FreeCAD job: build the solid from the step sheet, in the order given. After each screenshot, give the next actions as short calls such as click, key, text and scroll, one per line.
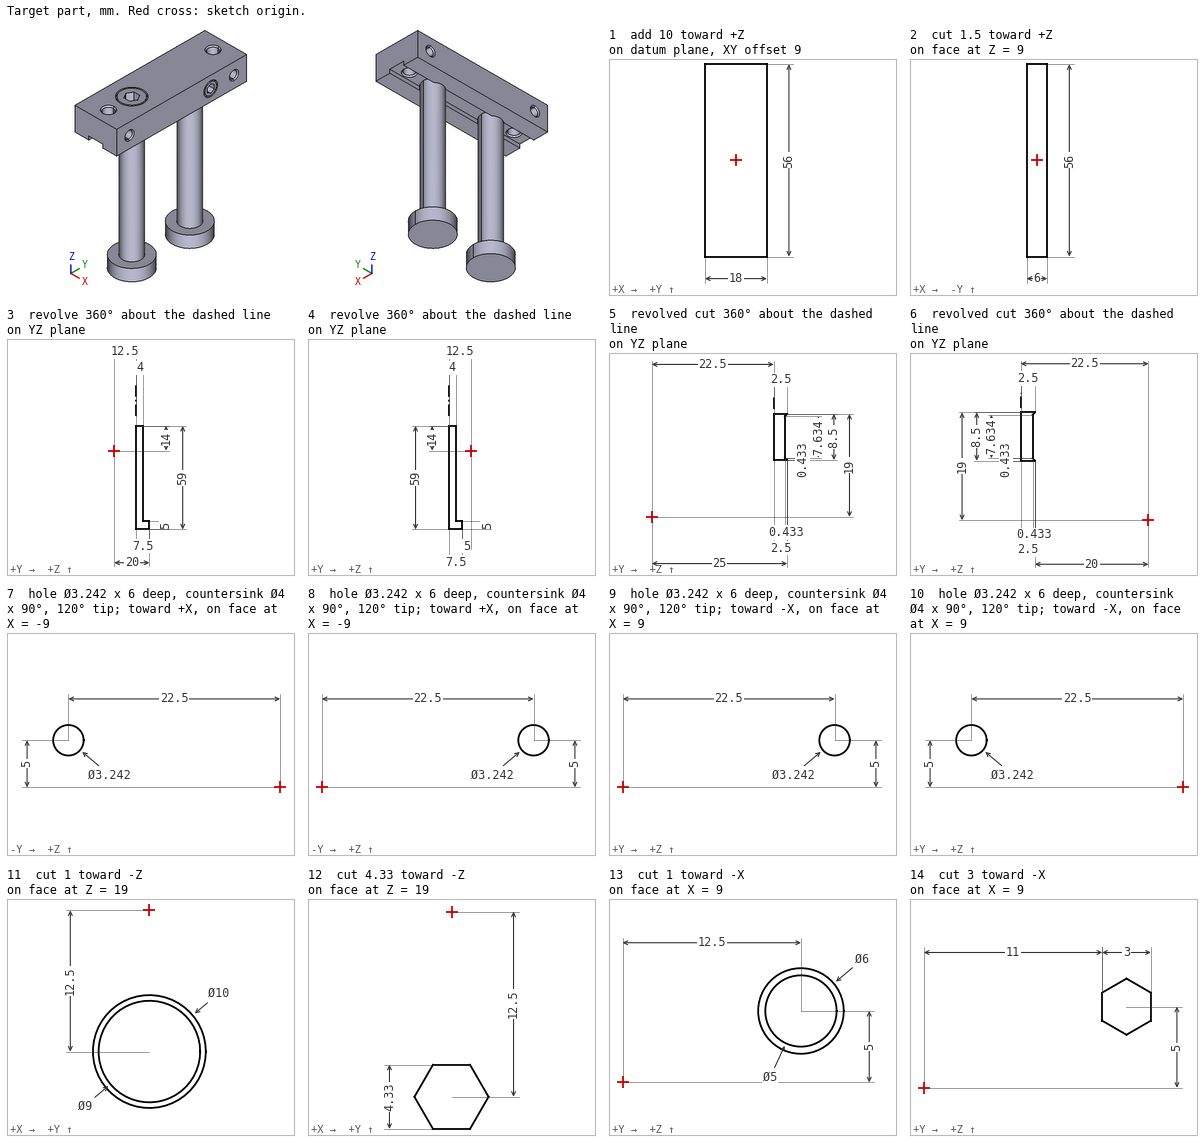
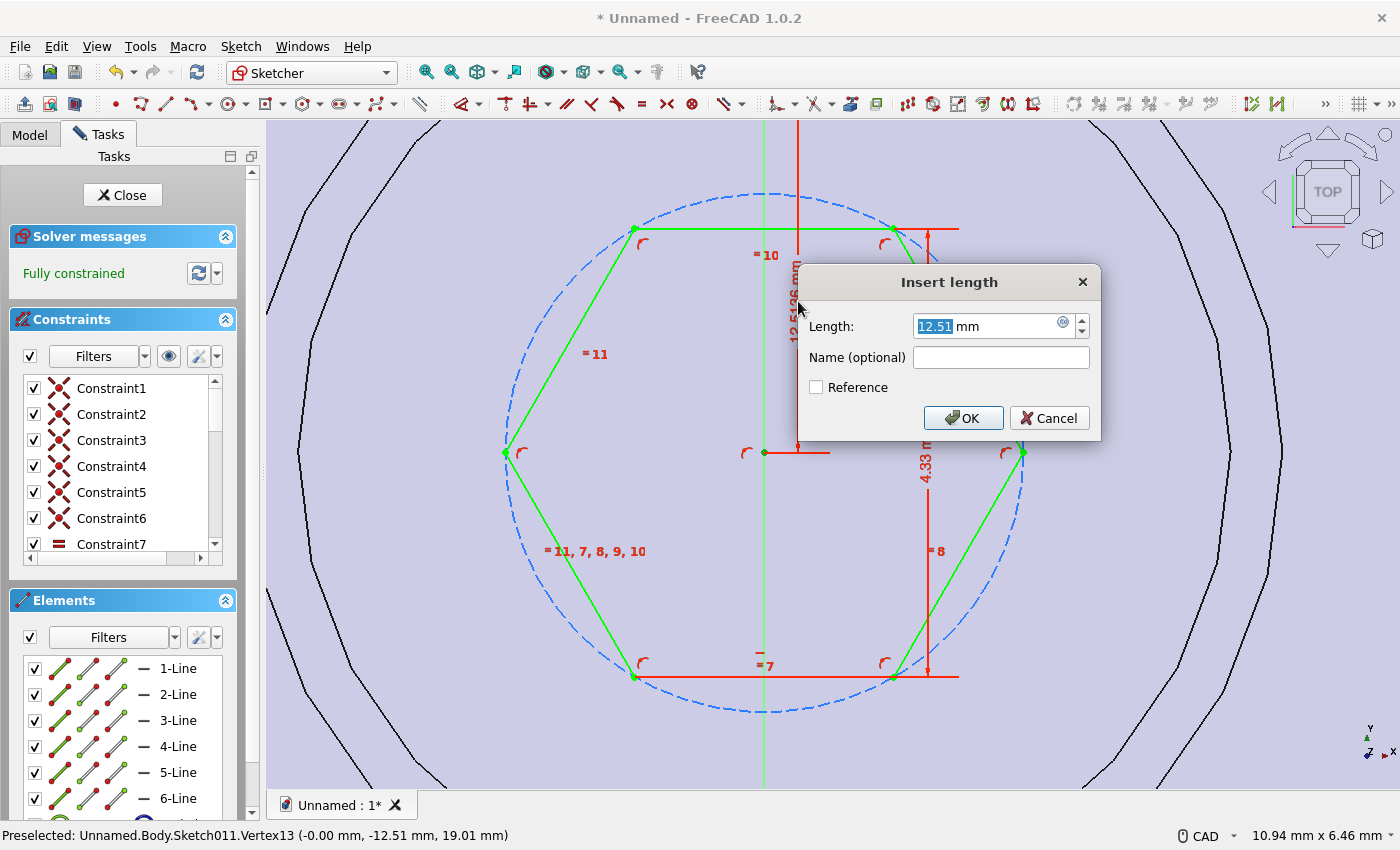
text(12.5)
key(Return)
key(Escape)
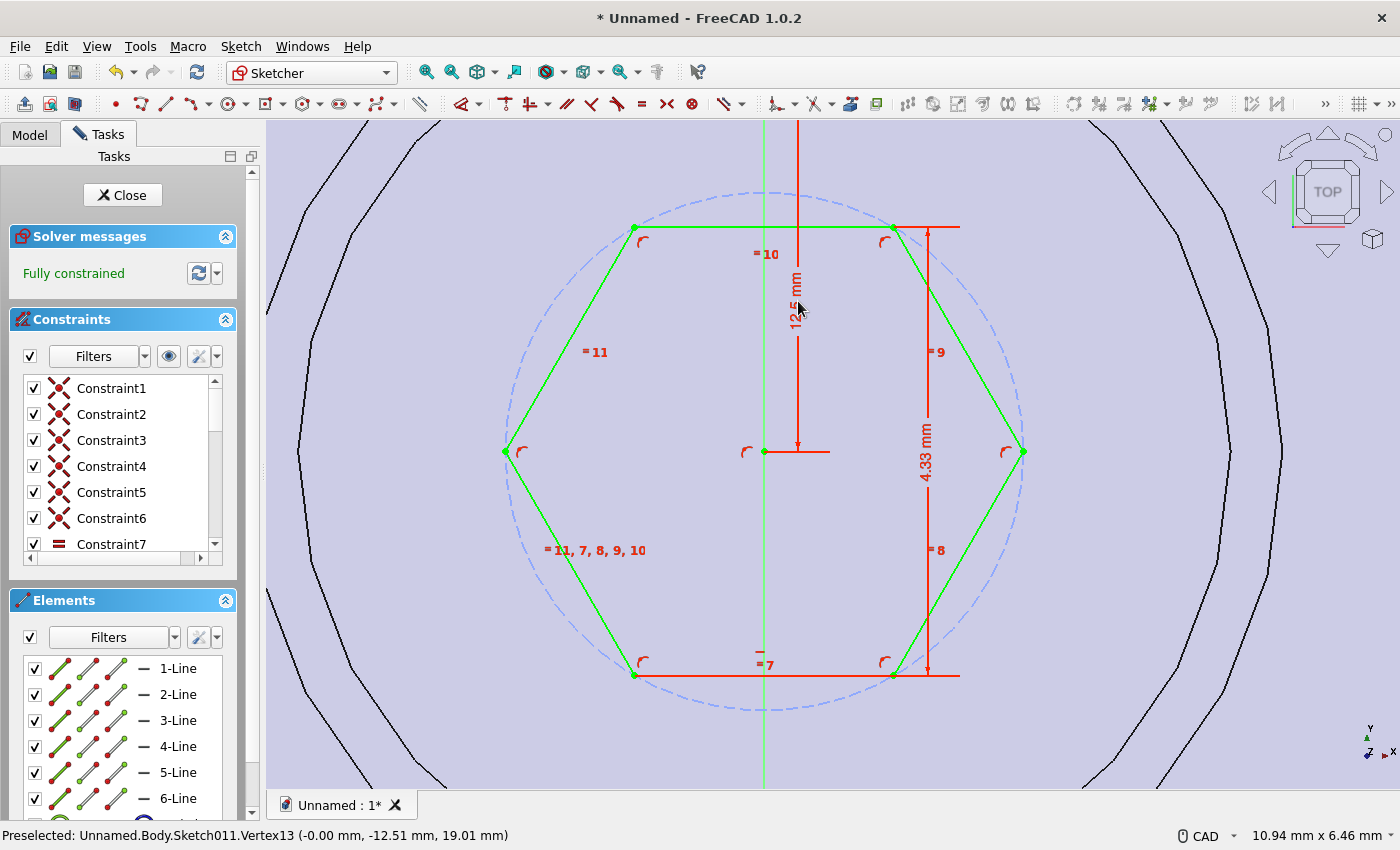
click(123, 195)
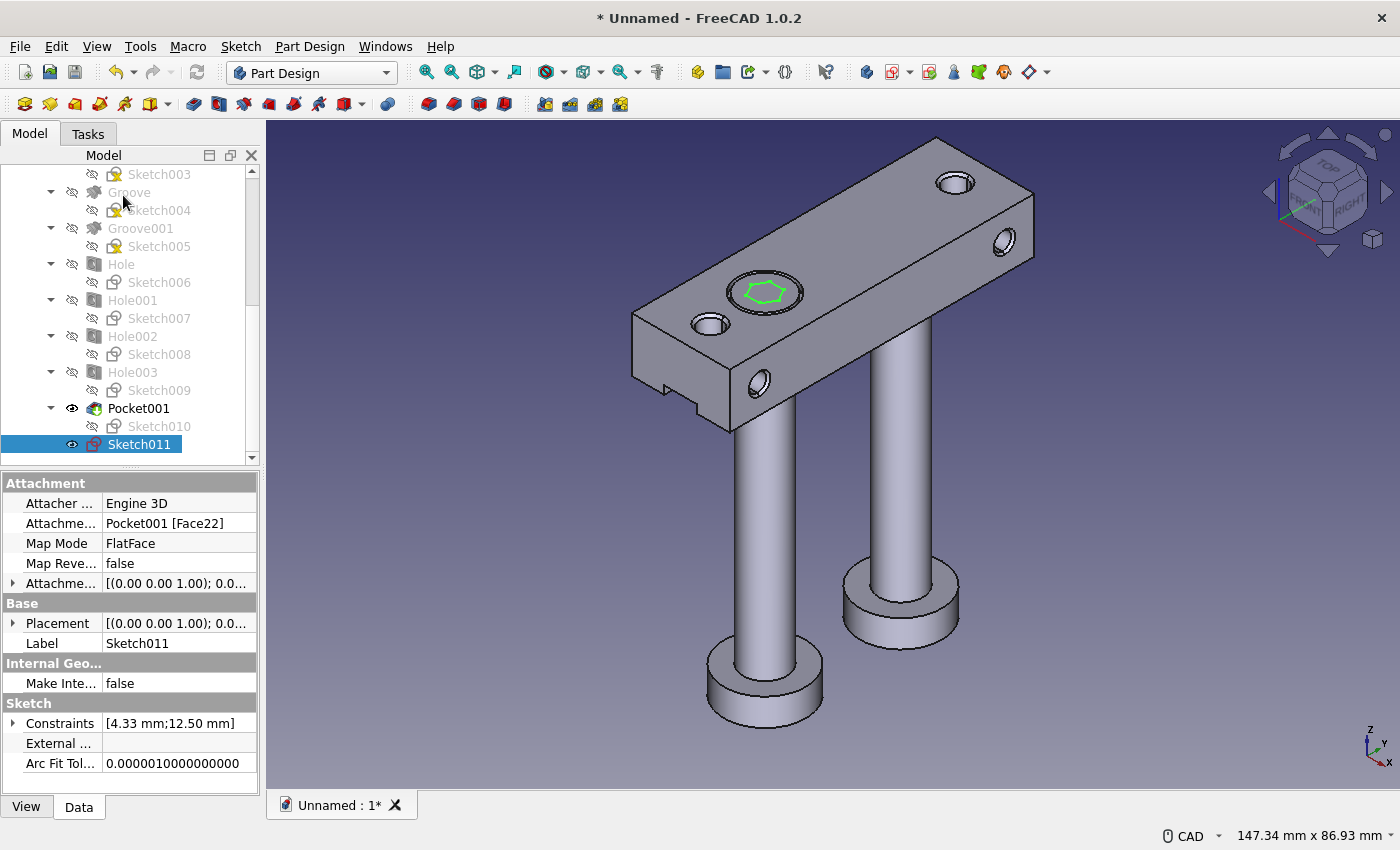
click(194, 104)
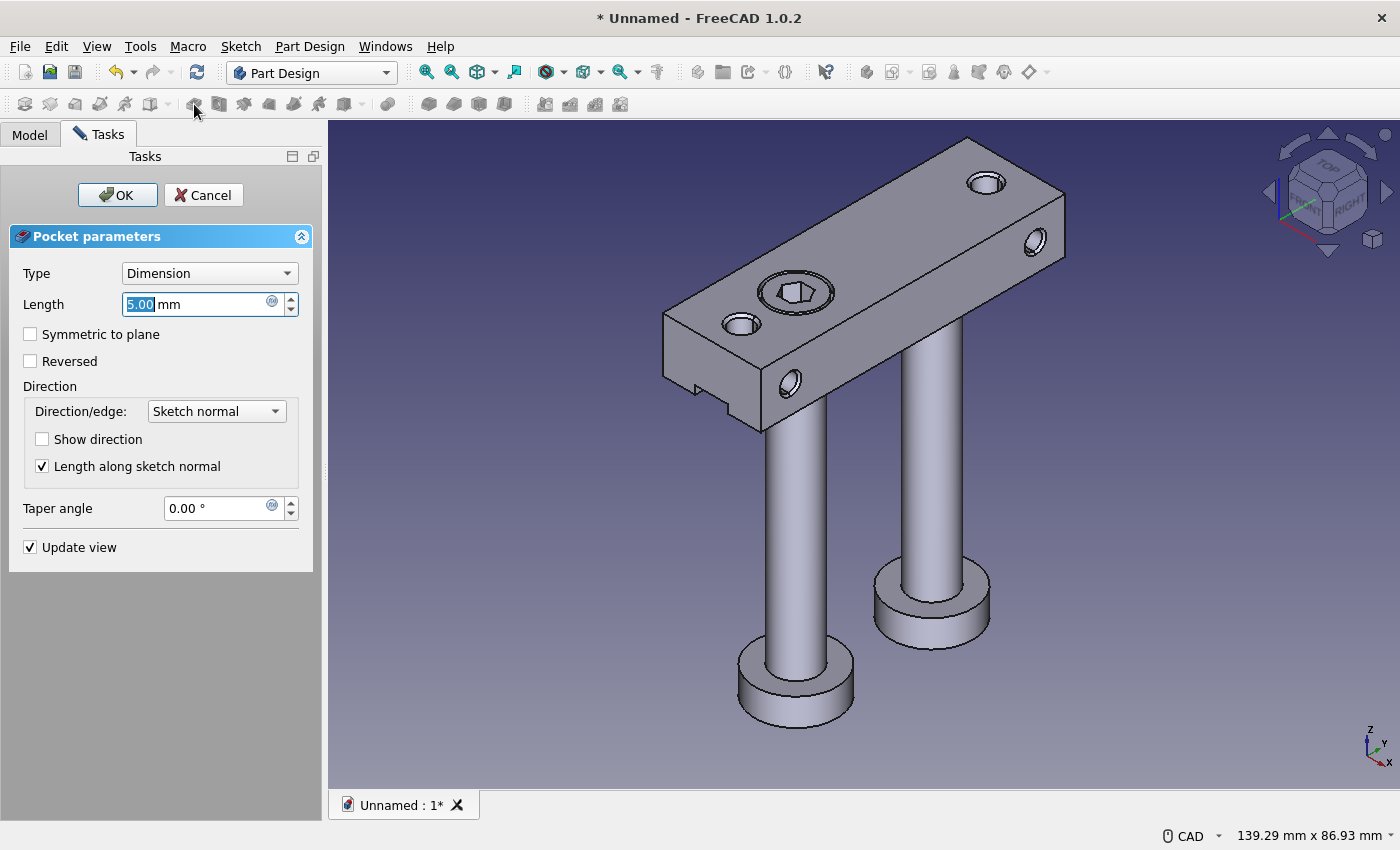
text(4.33)
key(Tab)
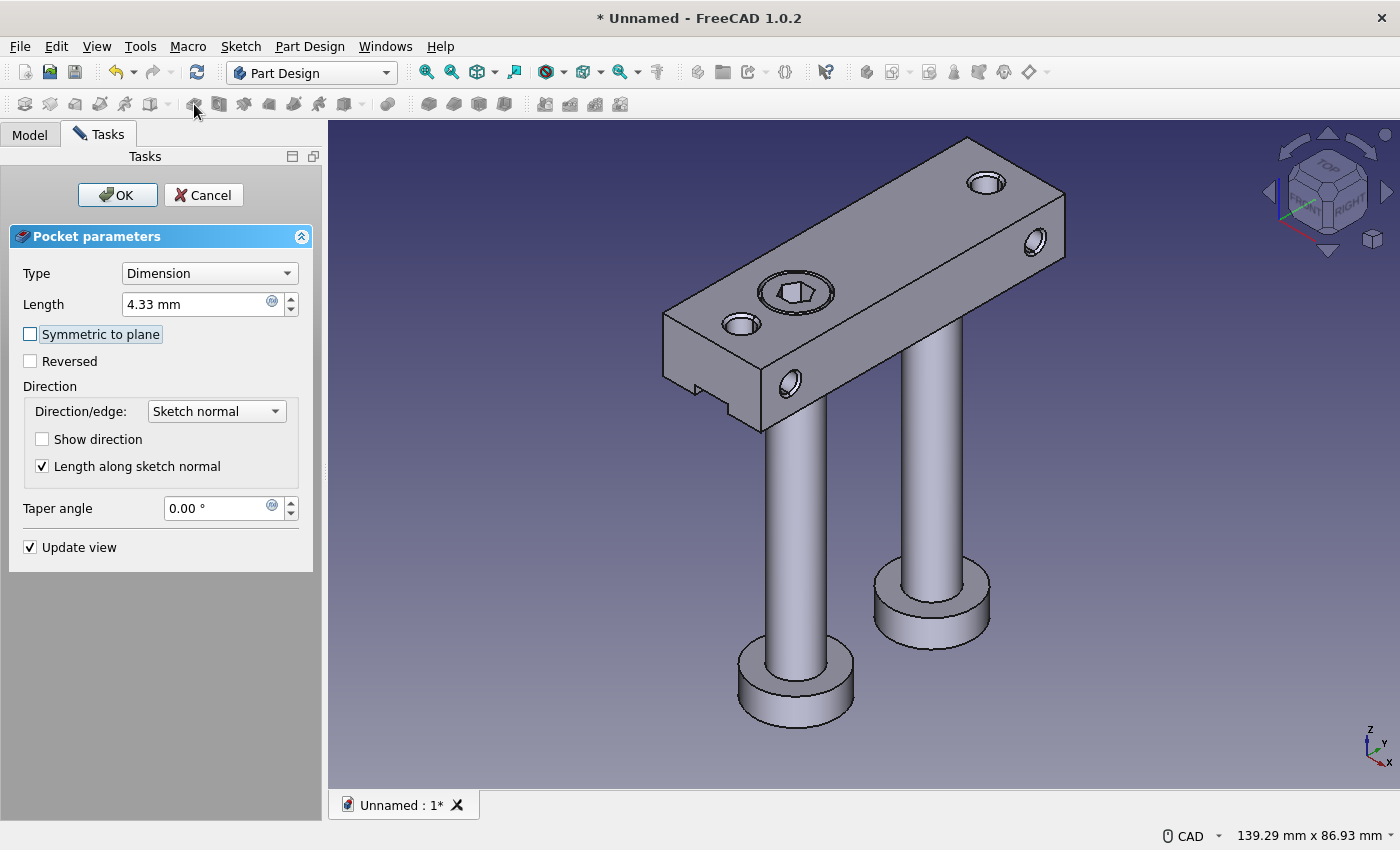
click(118, 195)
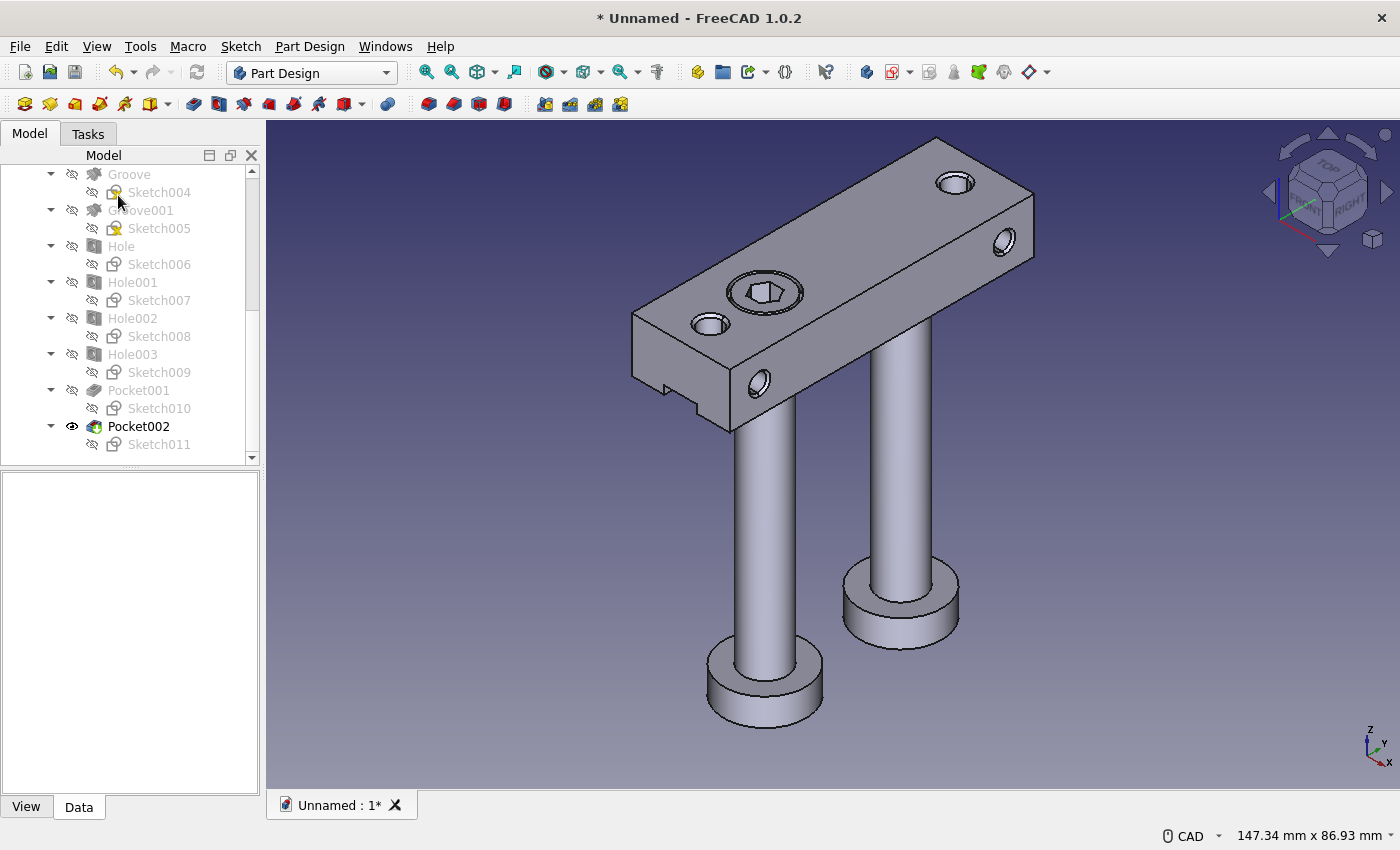
click(926, 287)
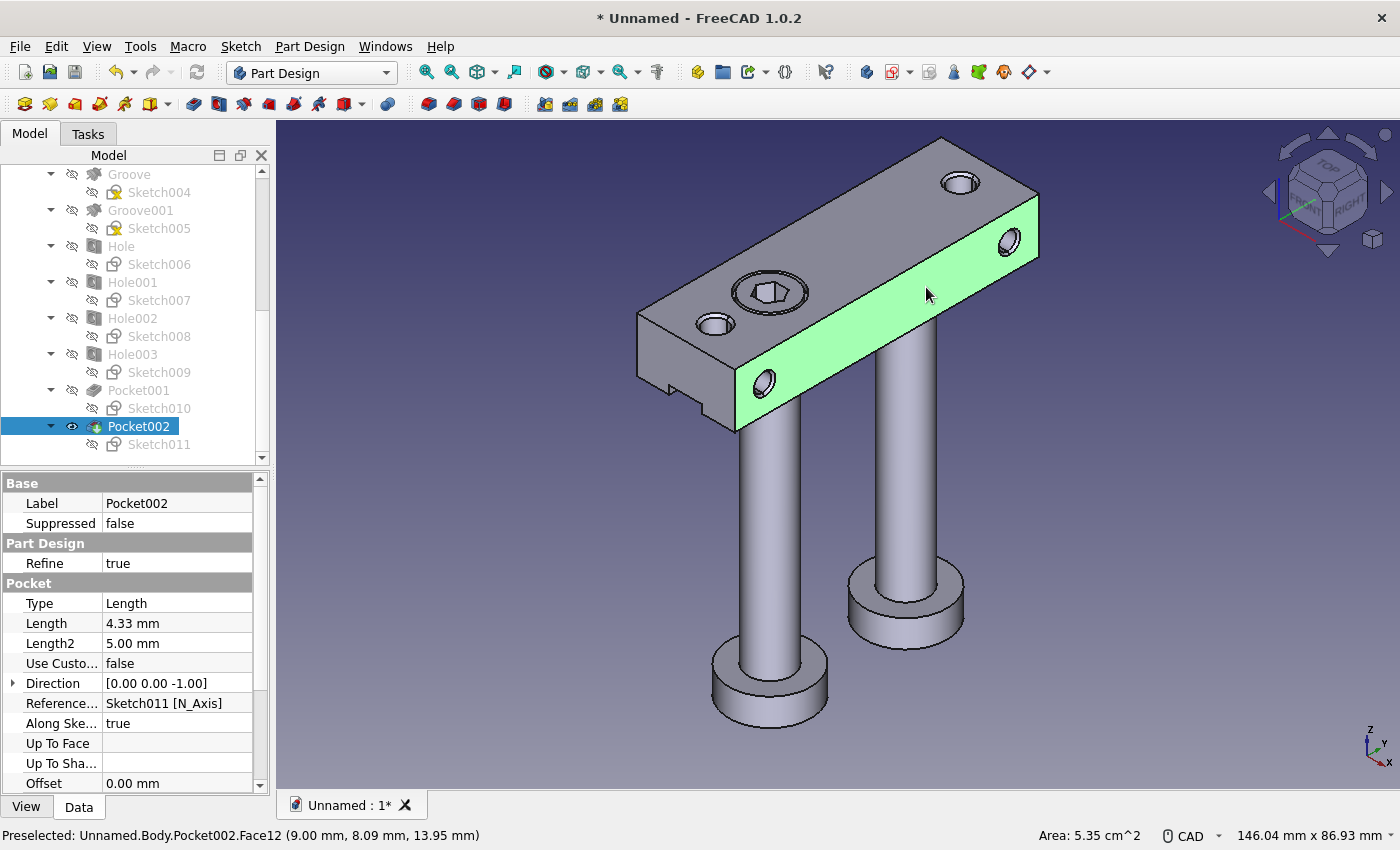
click(892, 72)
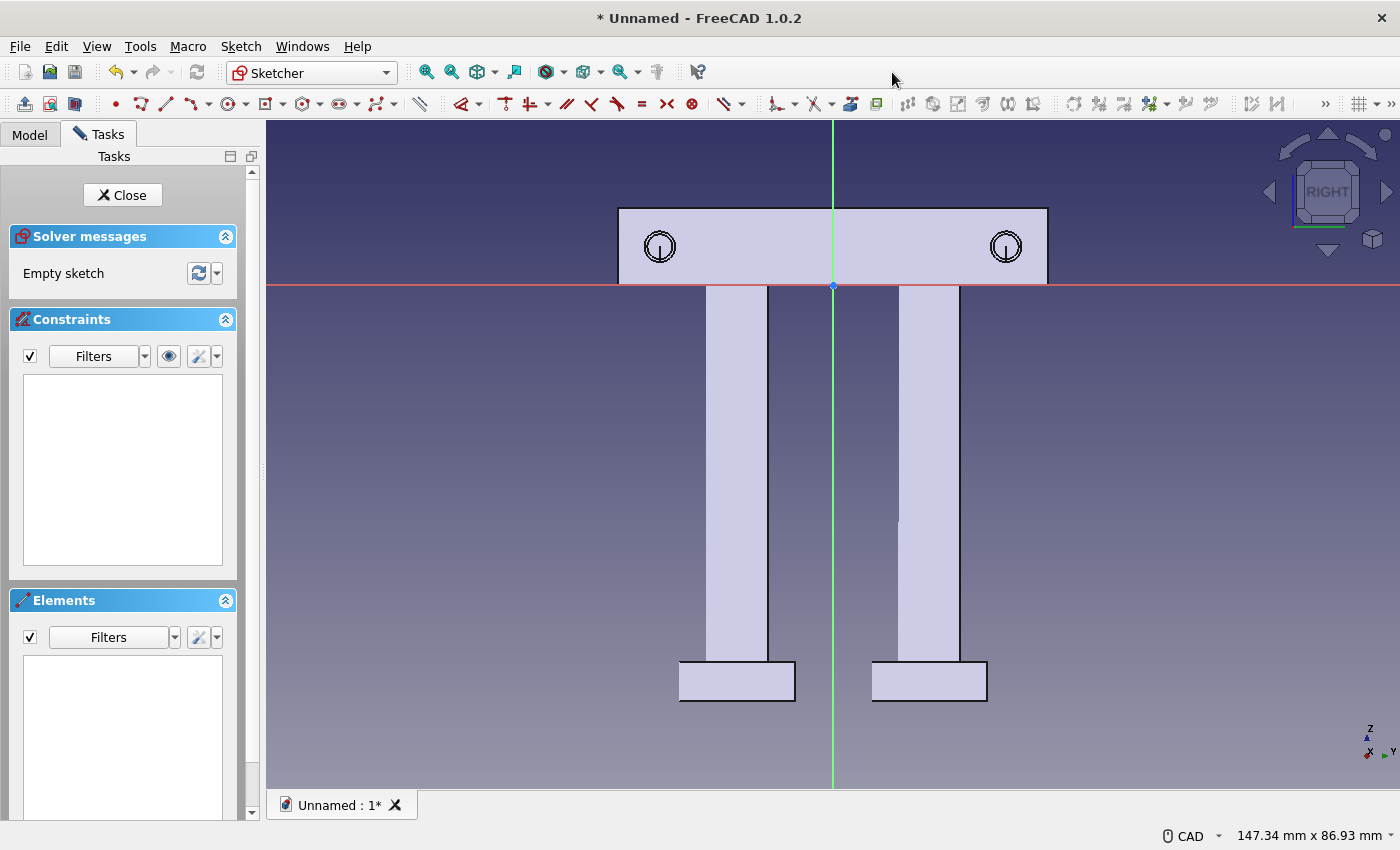
scroll(950, 221, up, 11)